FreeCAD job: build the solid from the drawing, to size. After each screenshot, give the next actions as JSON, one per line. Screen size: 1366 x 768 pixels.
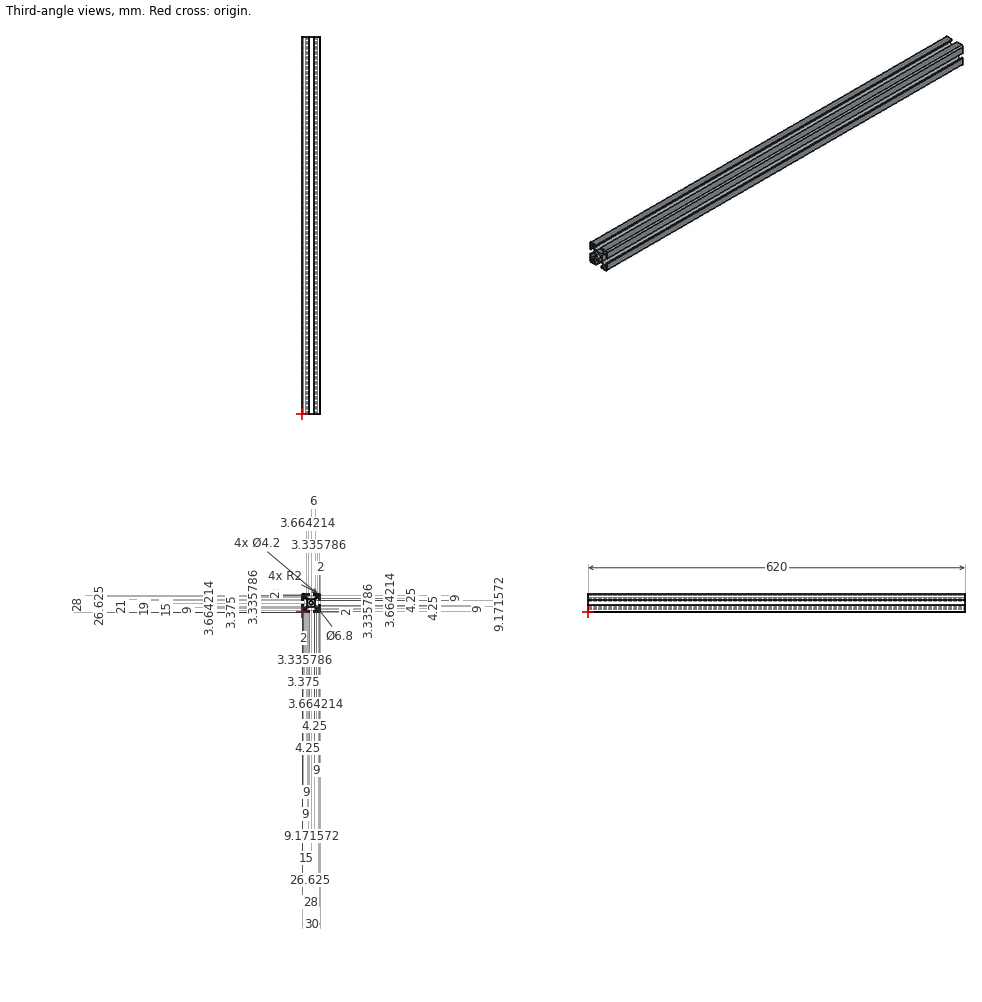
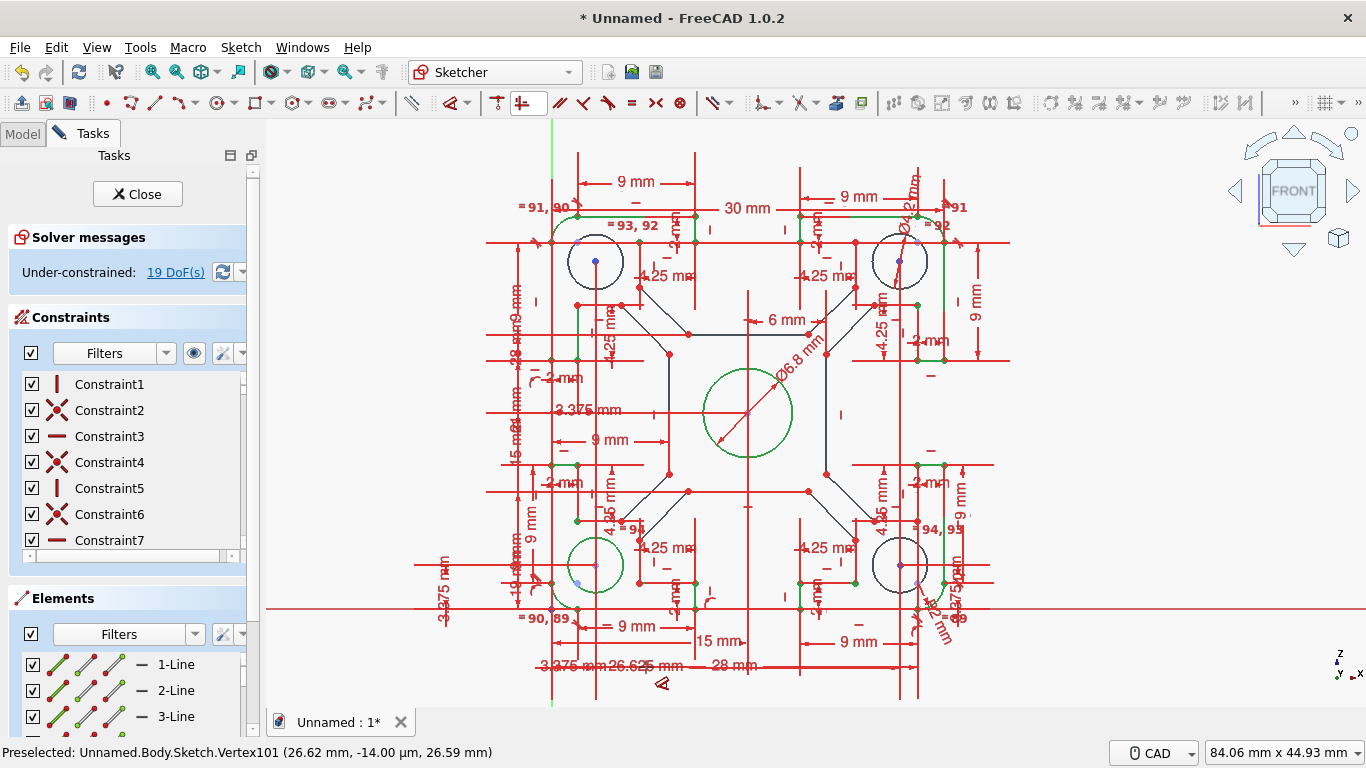
{"action": "left_click", "coordinate": [900, 261]}
{"action": "left_click", "coordinate": [934, 435]}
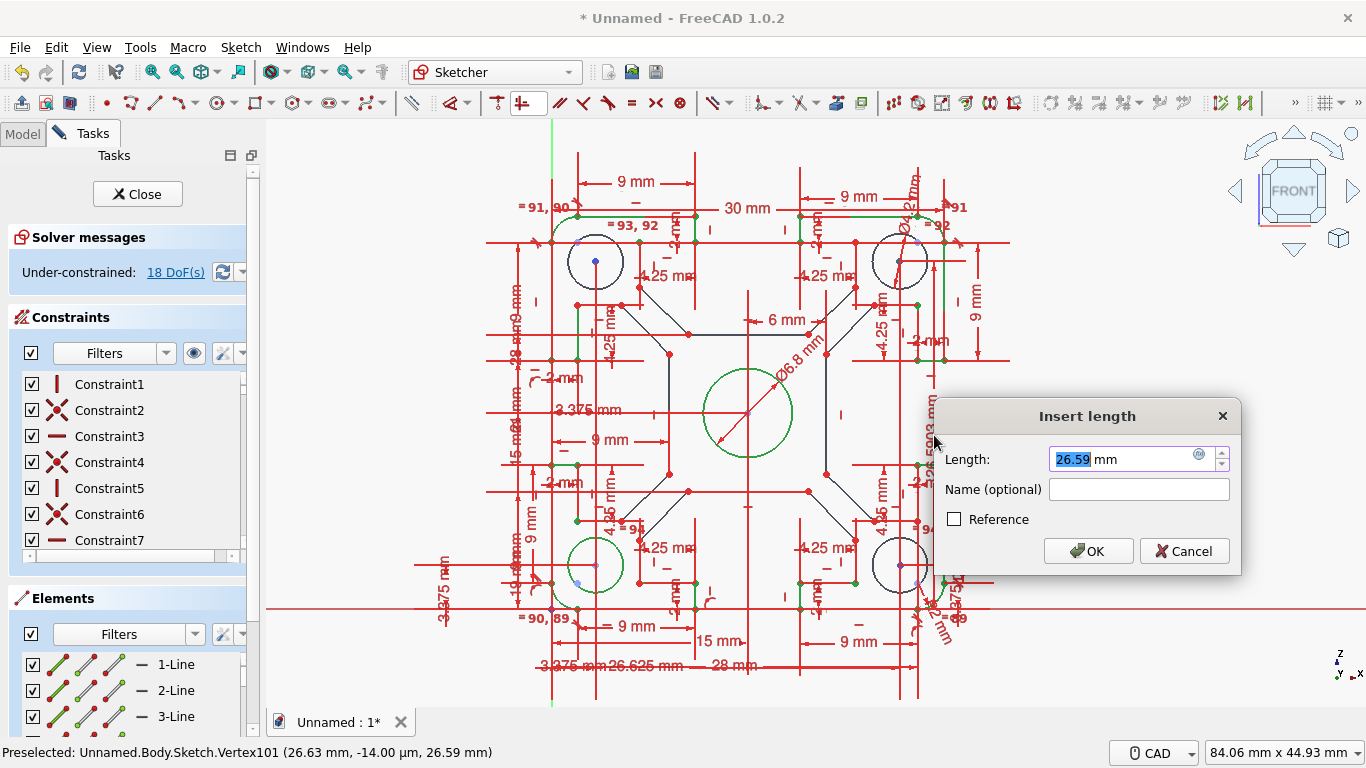
{"action": "type", "text": "26.625"}
{"action": "key", "text": "Return"}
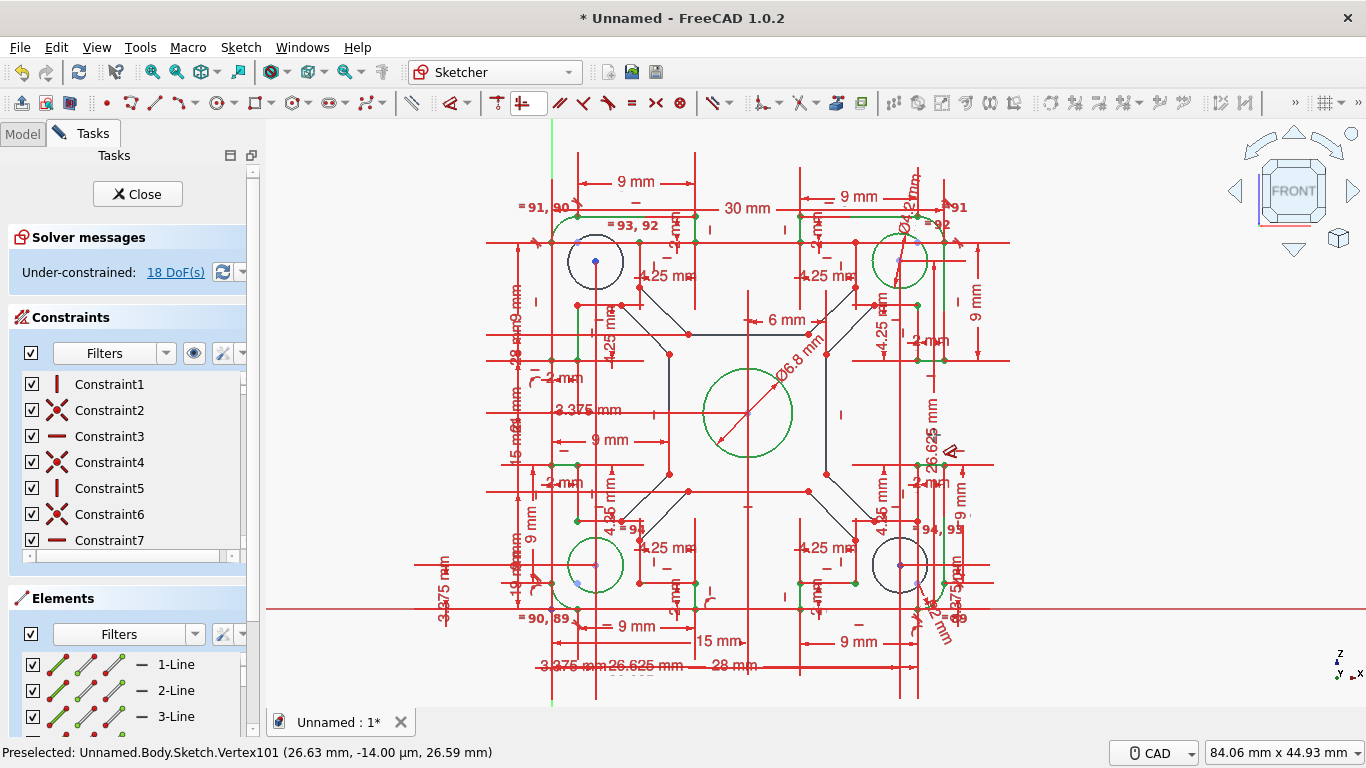
{"action": "left_click", "coordinate": [596, 262]}
{"action": "left_click", "coordinate": [630, 356]}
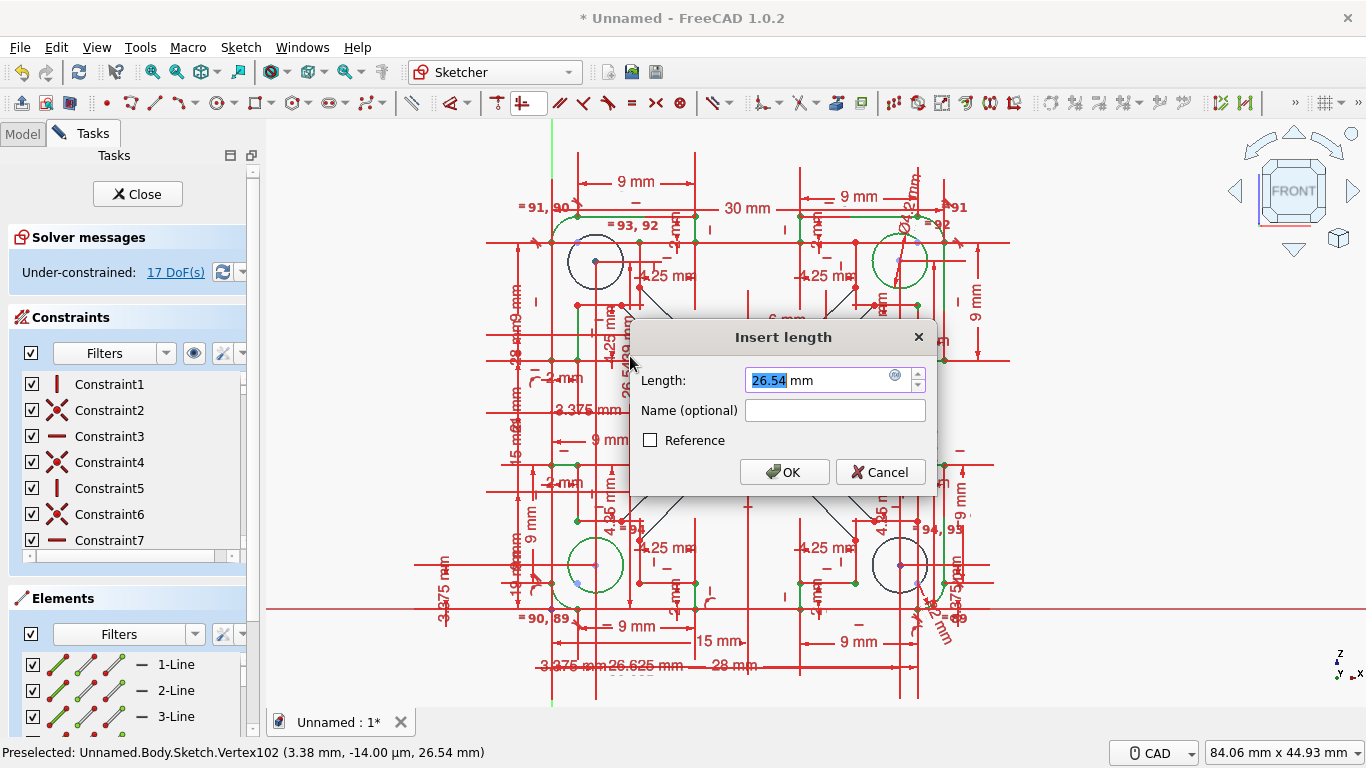
{"action": "type", "text": "26.625"}
{"action": "key", "text": "Return"}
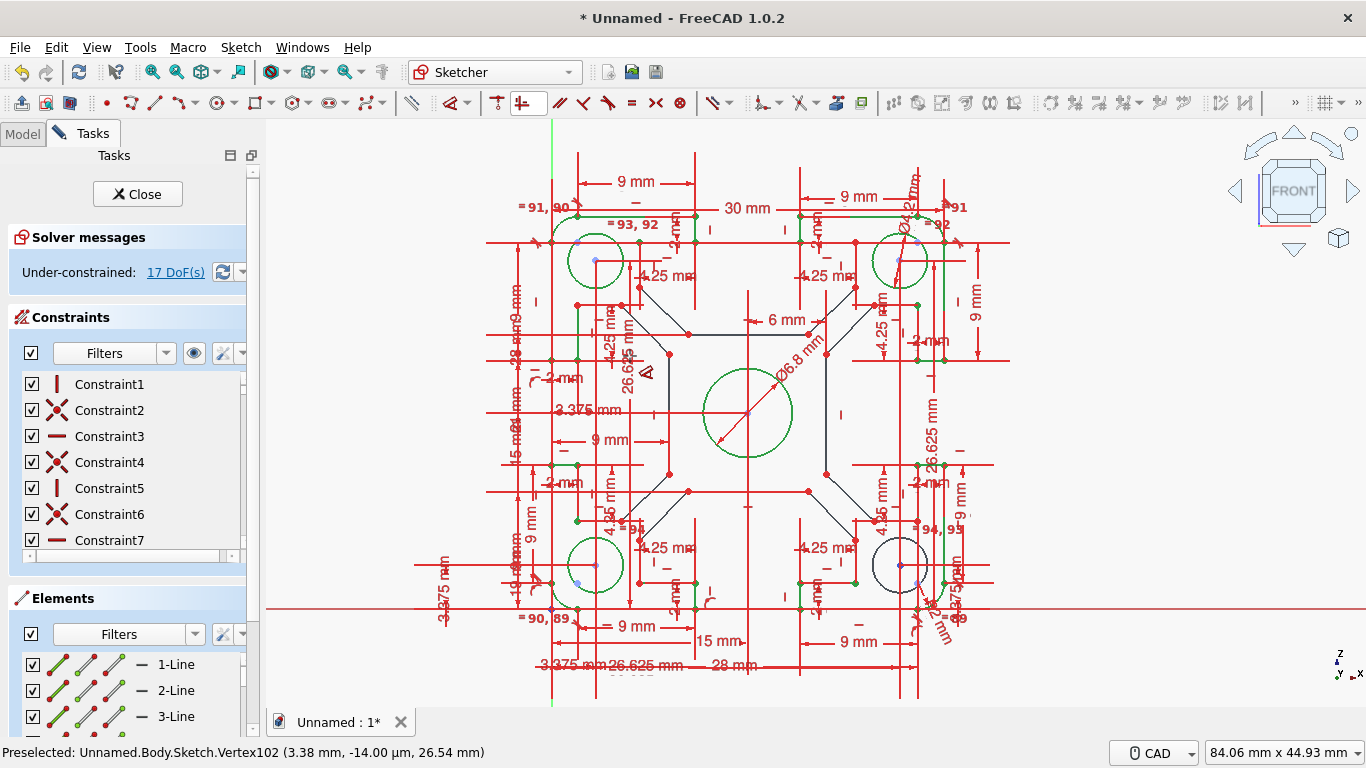
{"action": "left_click", "coordinate": [900, 565]}
{"action": "left_click", "coordinate": [806, 667]}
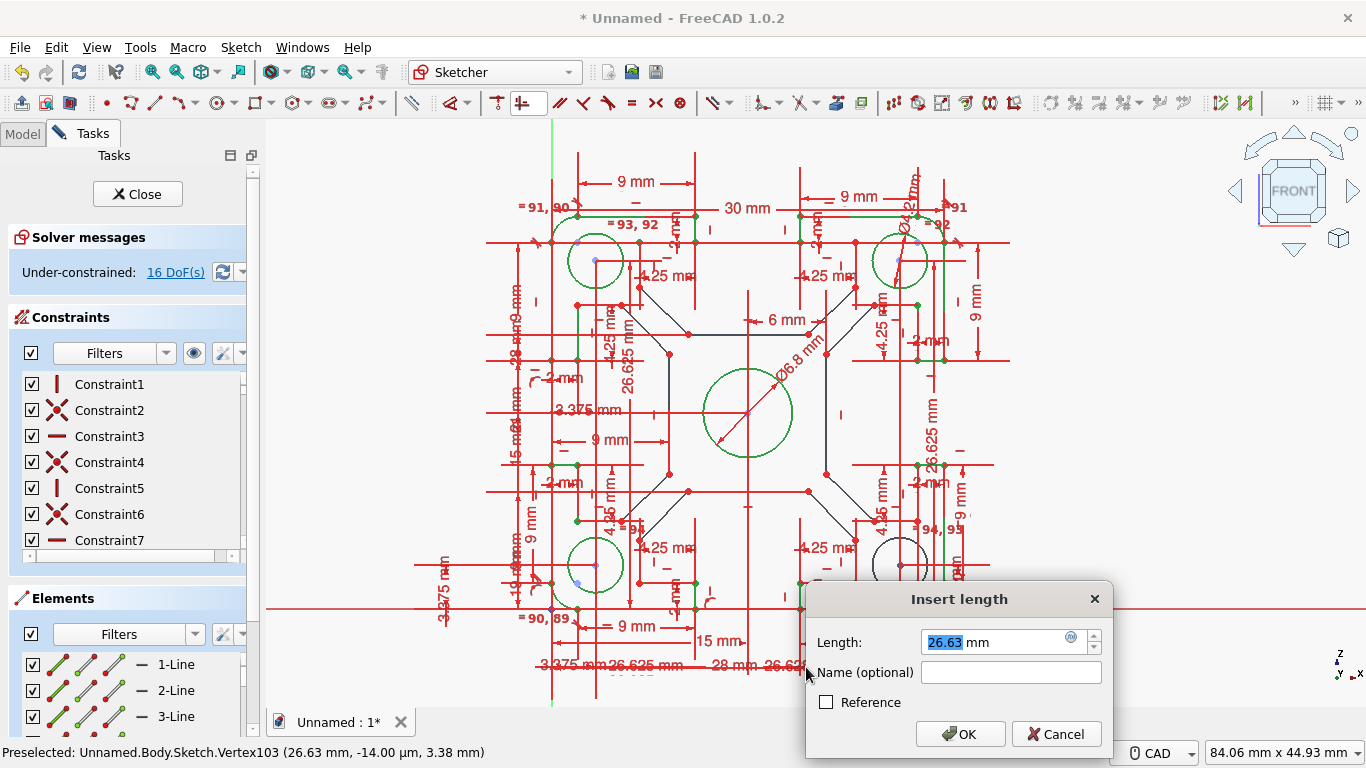
{"action": "type", "text": "26.625"}
{"action": "key", "text": "Return"}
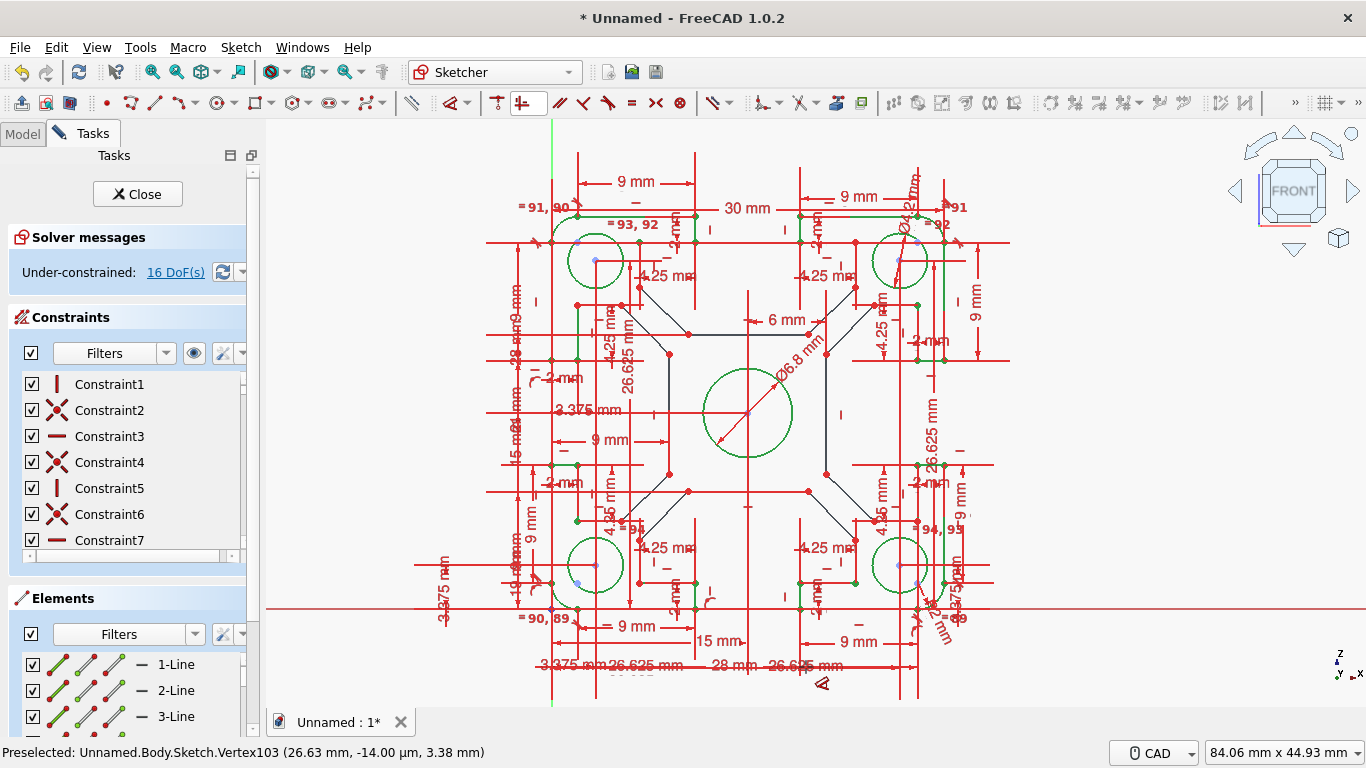
{"action": "left_click", "coordinate": [905, 305]}
{"action": "left_click", "coordinate": [906, 271]}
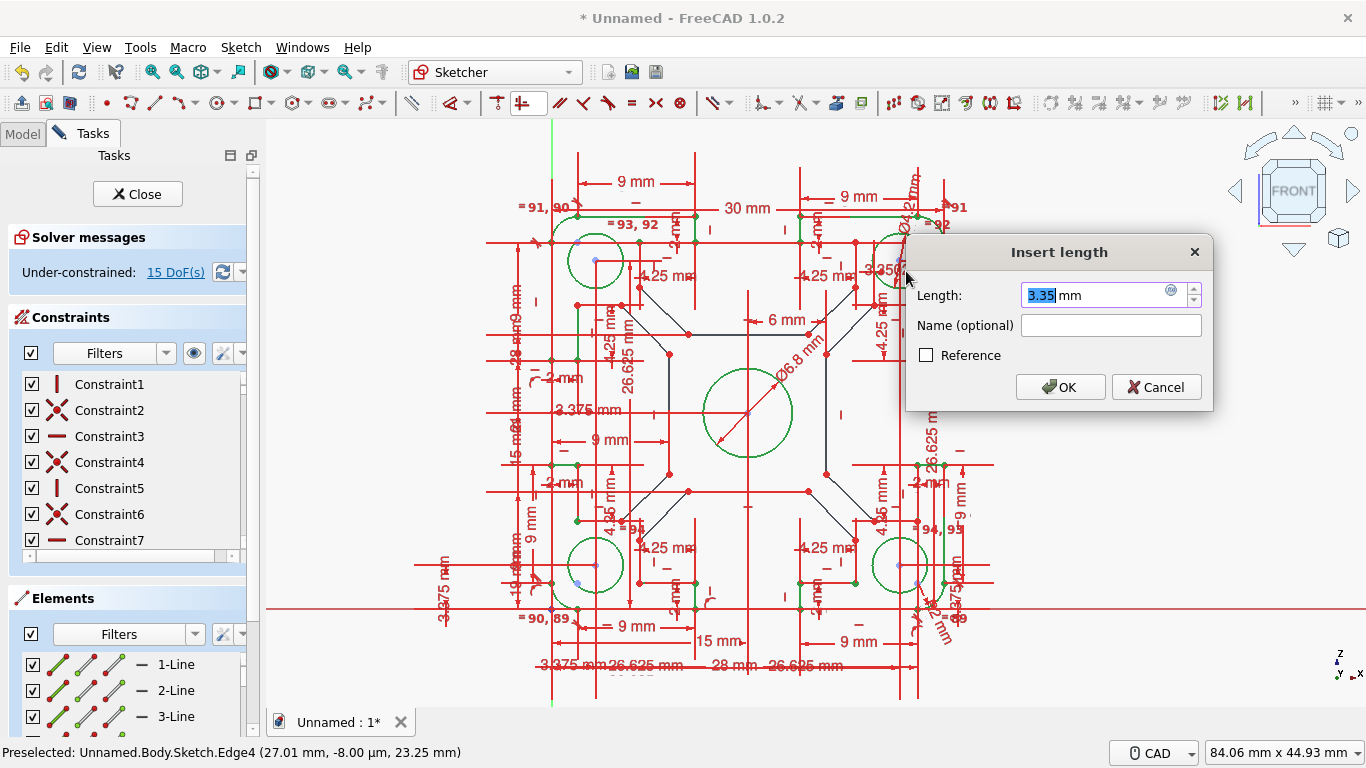
{"action": "type", "text": "3.335786"}
{"action": "key", "text": "Return"}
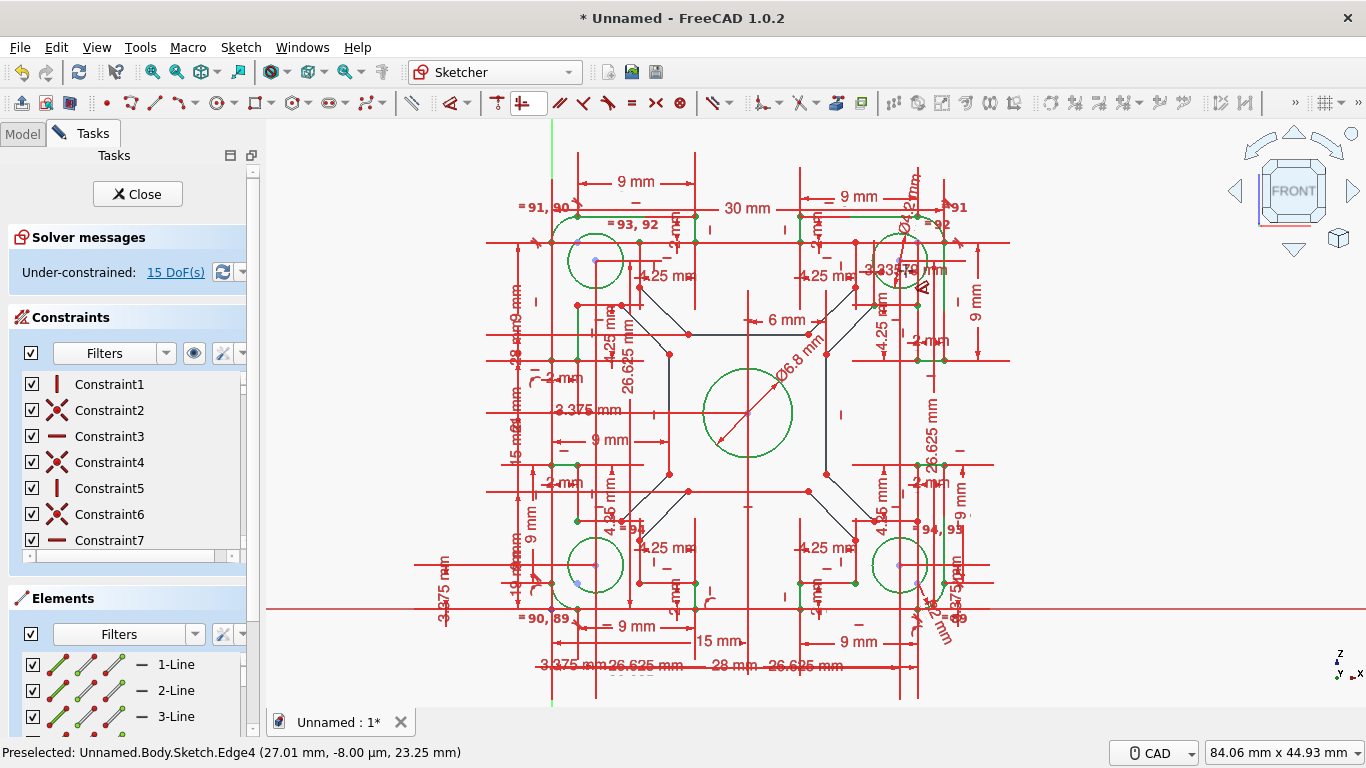
{"action": "left_click", "coordinate": [826, 391]}
{"action": "left_click", "coordinate": [860, 415]}